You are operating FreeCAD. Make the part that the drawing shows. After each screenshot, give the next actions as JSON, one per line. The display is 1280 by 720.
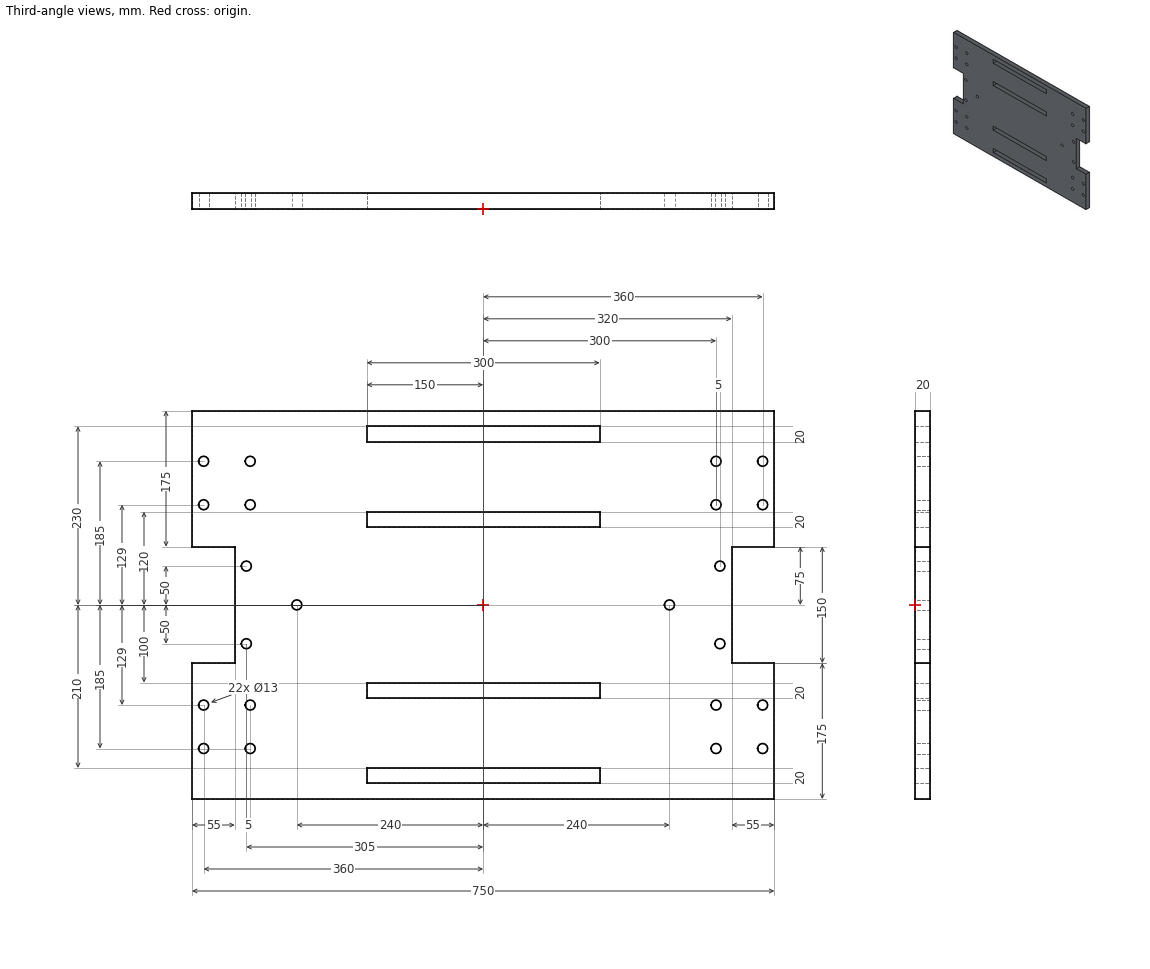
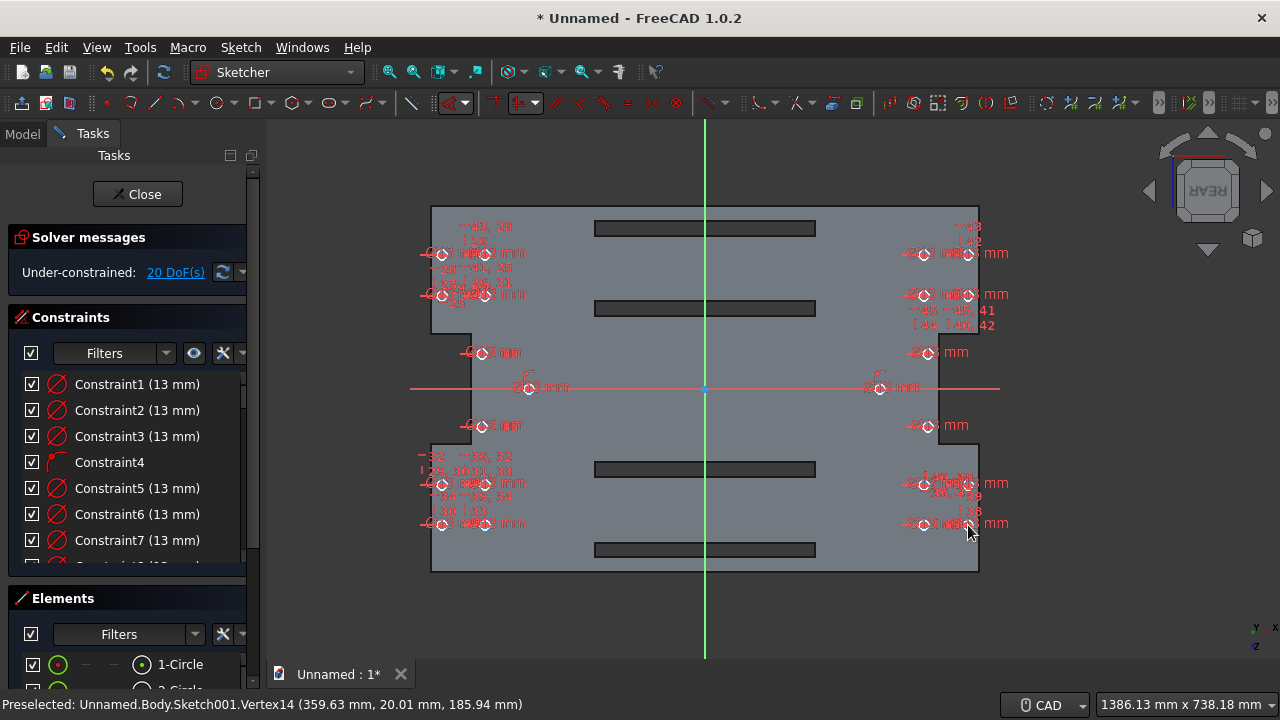
{"action": "left_click", "coordinate": [924, 525]}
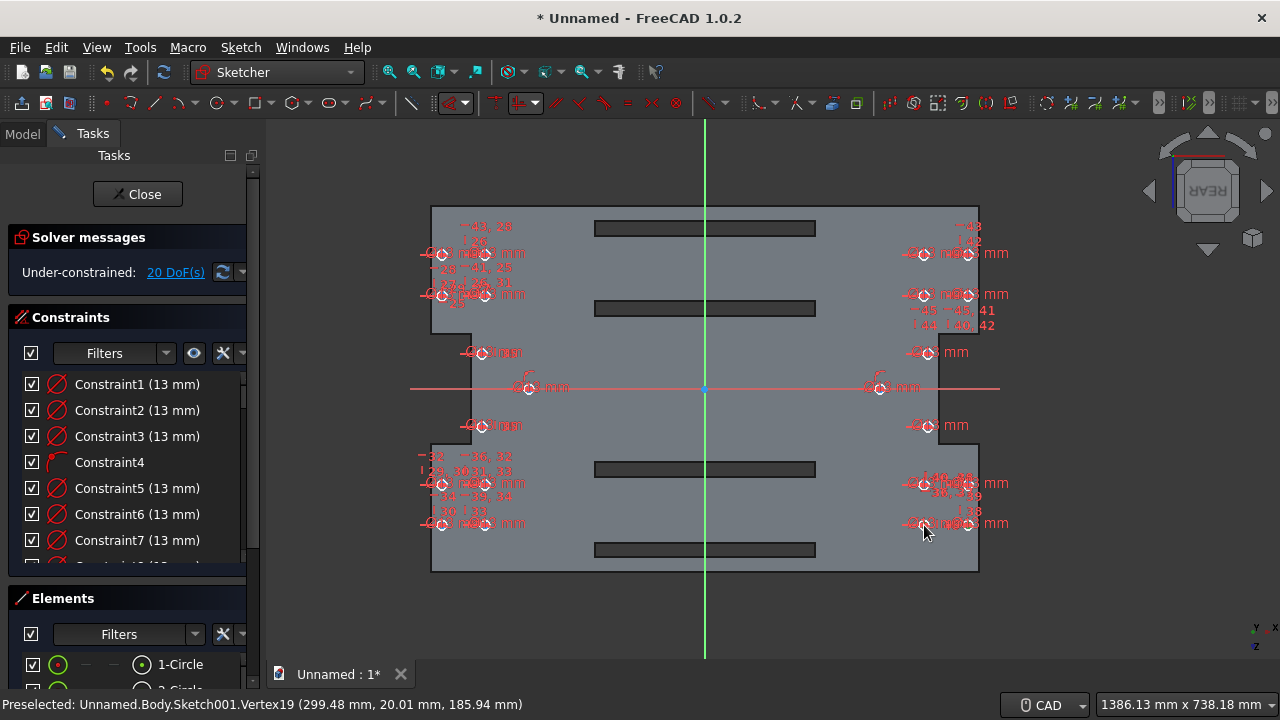
{"action": "left_click", "coordinate": [538, 104]}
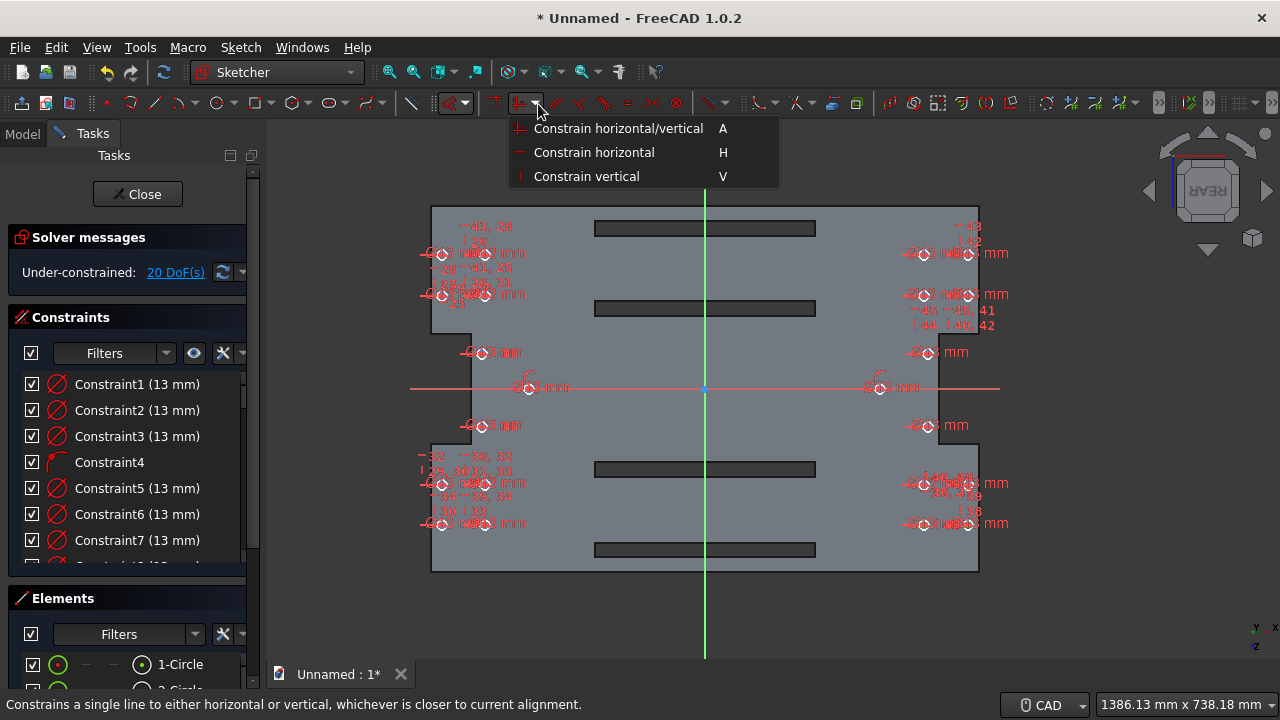
{"action": "left_click", "coordinate": [644, 152]}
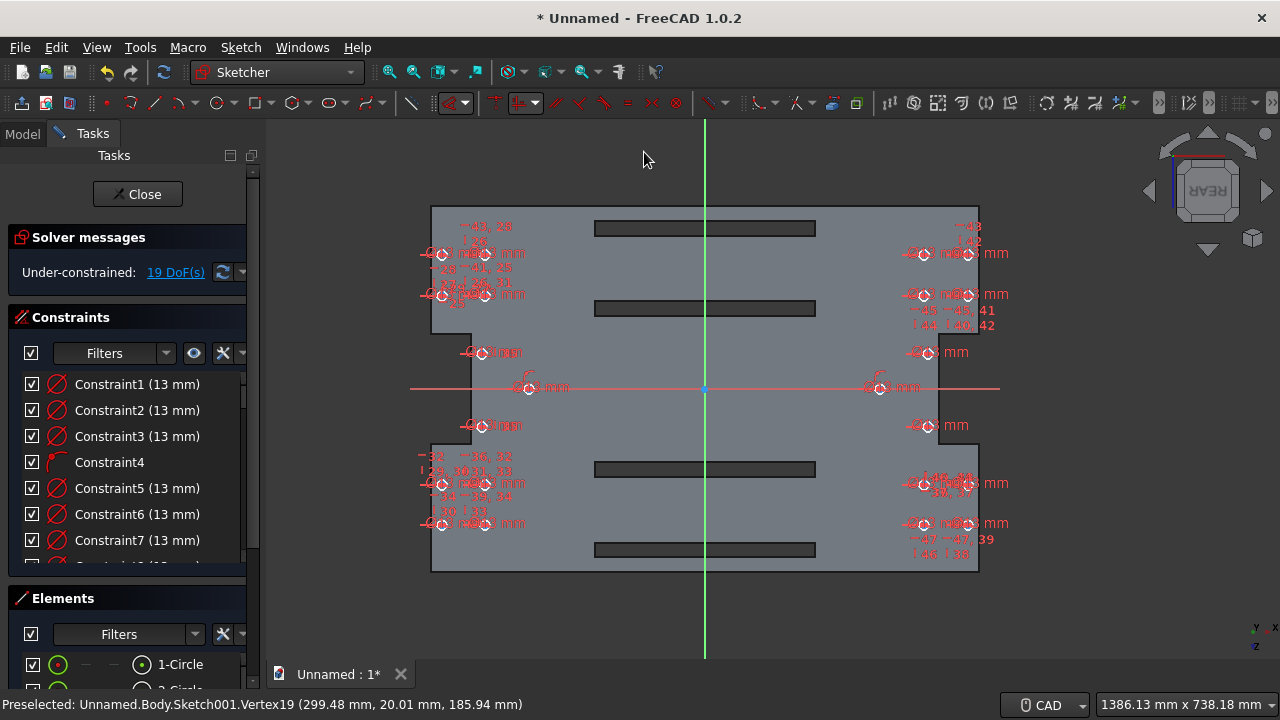
{"action": "left_click", "coordinate": [924, 296]}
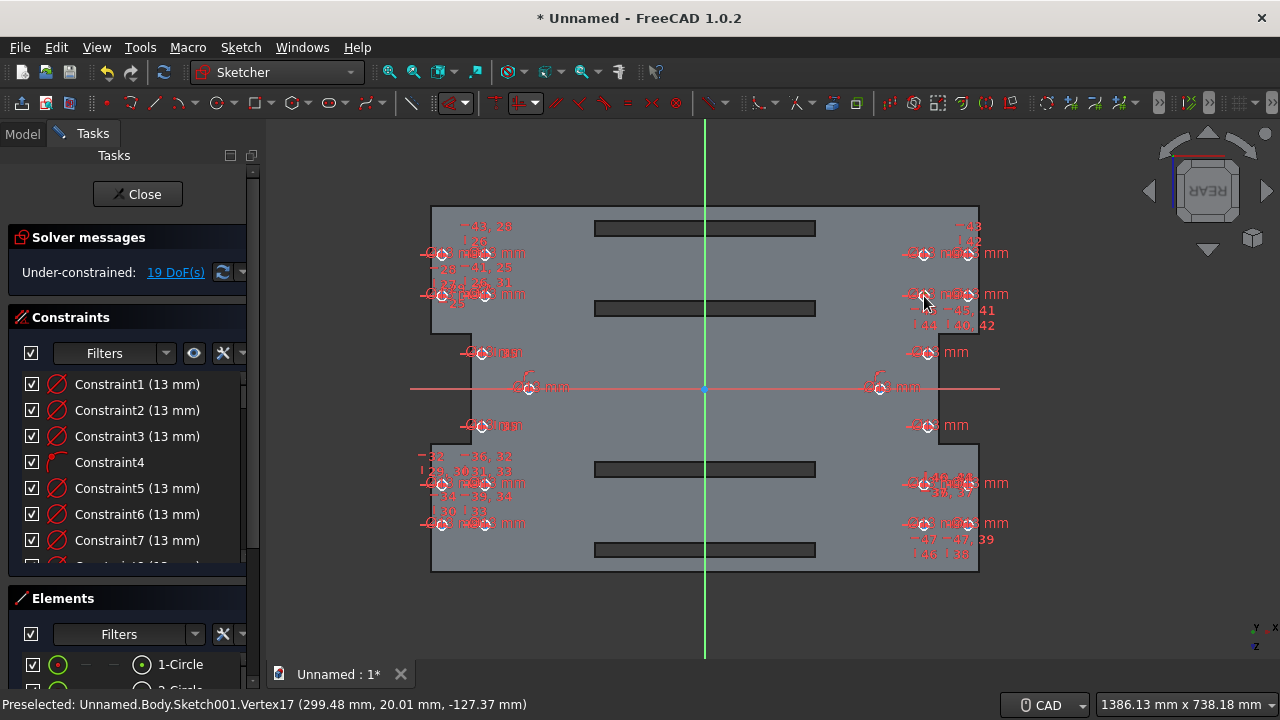
{"action": "left_click", "coordinate": [924, 255]}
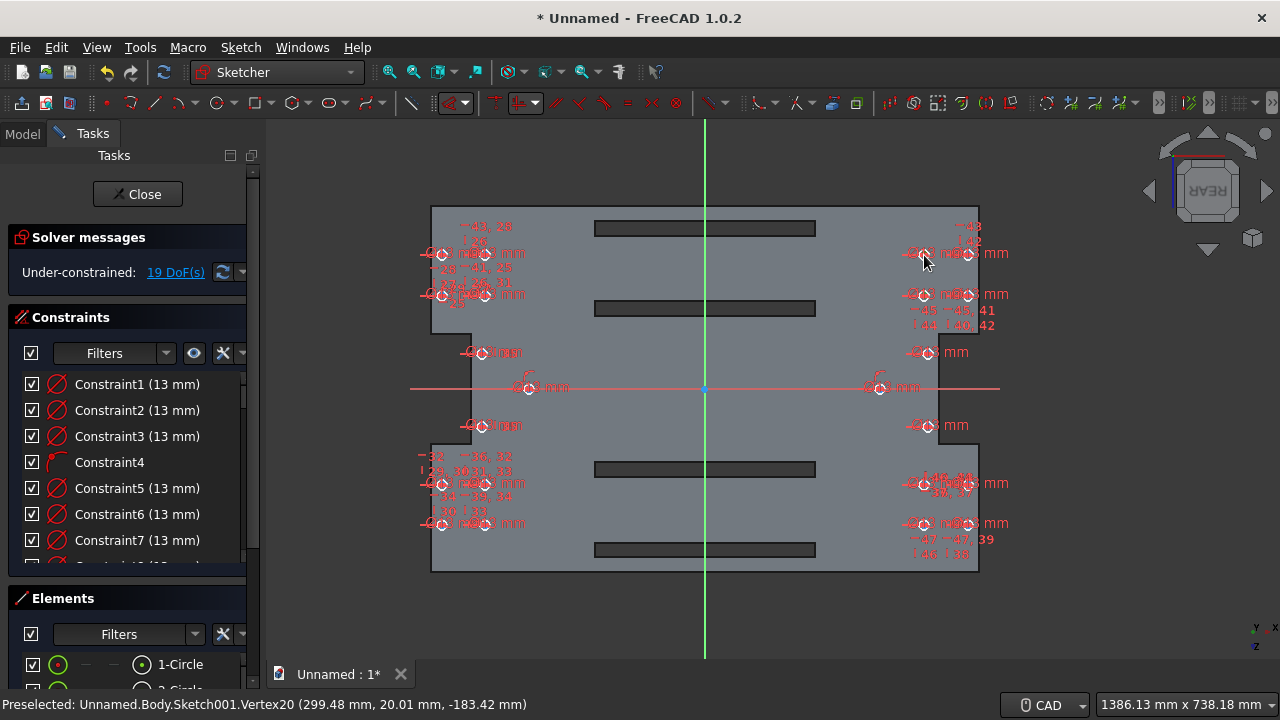
{"action": "left_click", "coordinate": [538, 104]}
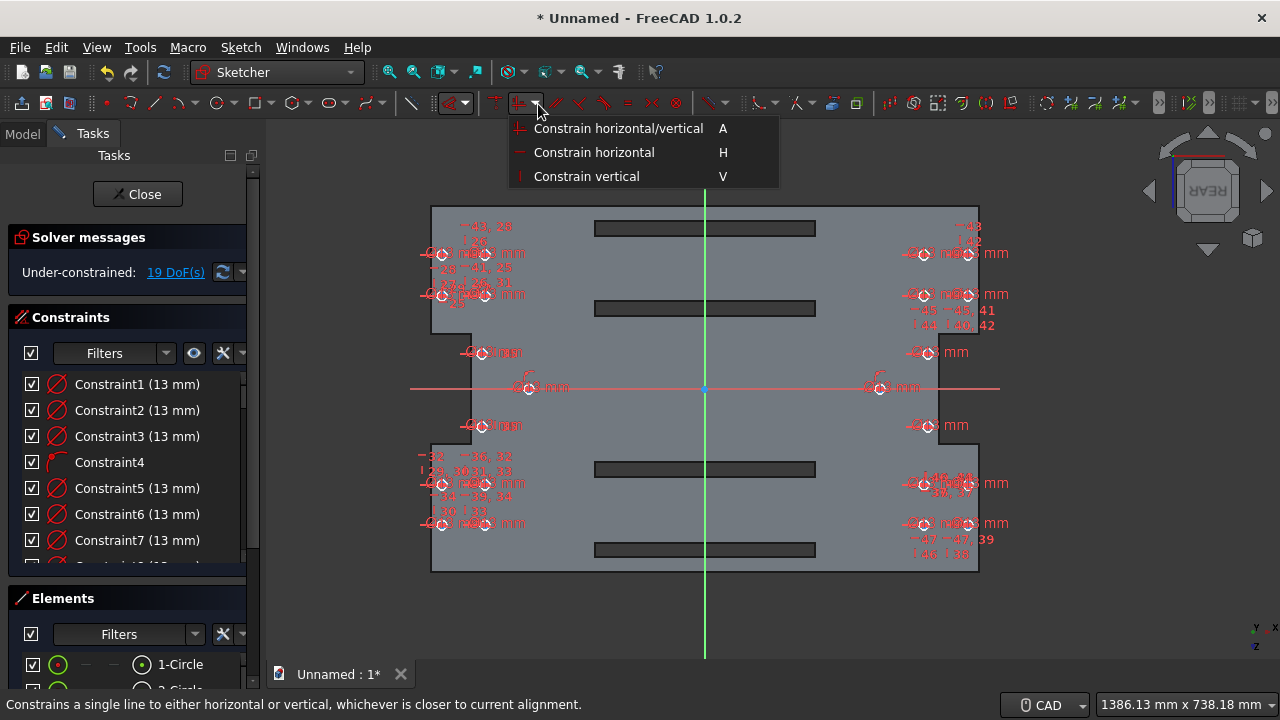
{"action": "left_click", "coordinate": [644, 176]}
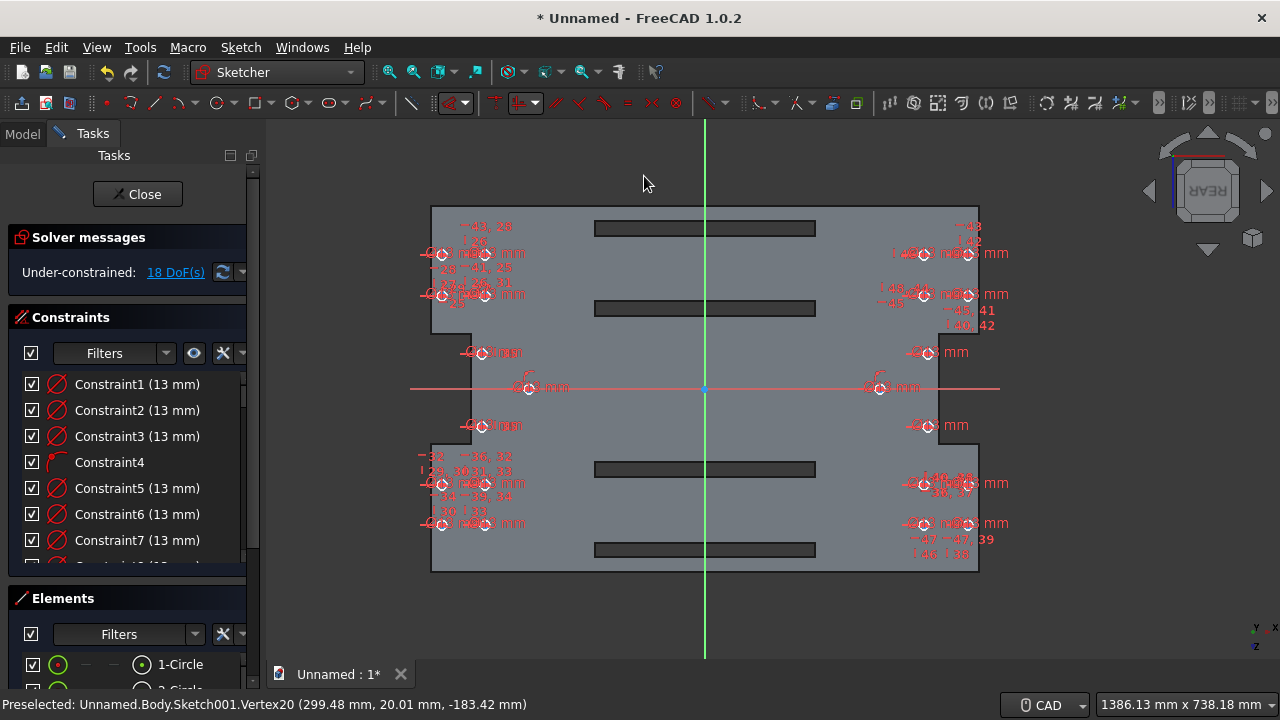
{"action": "left_click", "coordinate": [968, 255]}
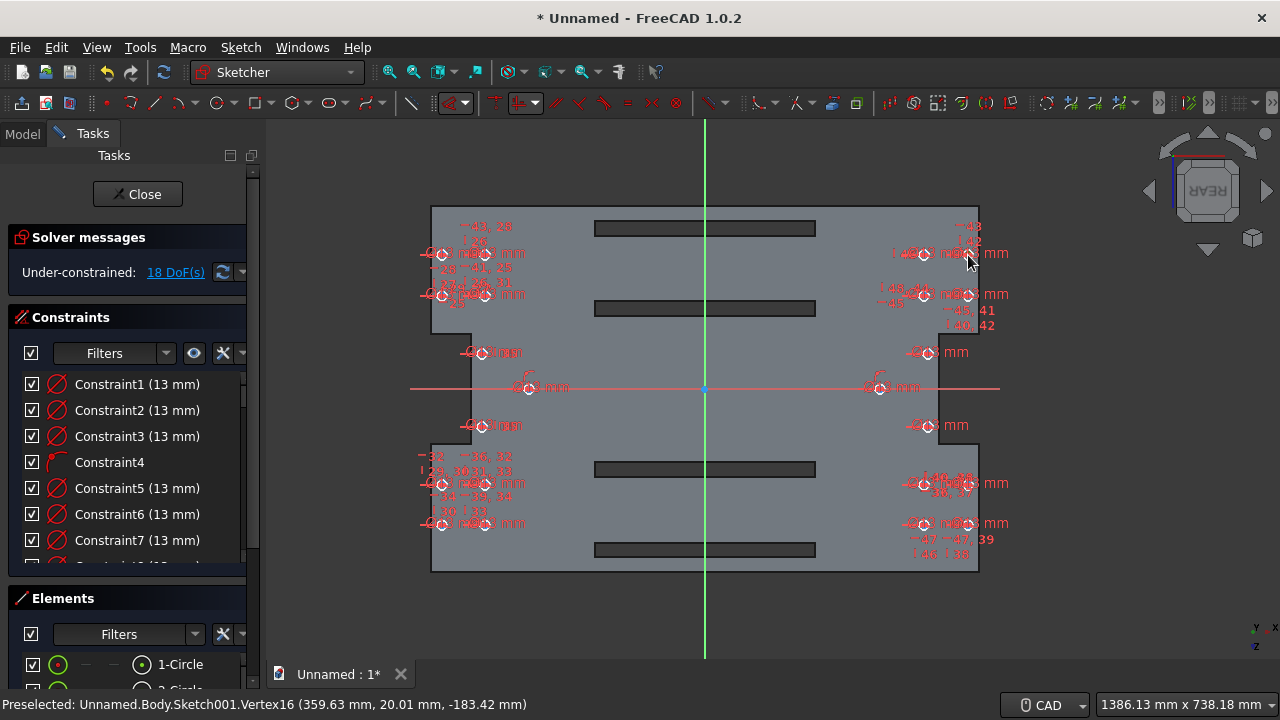
{"action": "left_click", "coordinate": [924, 255]}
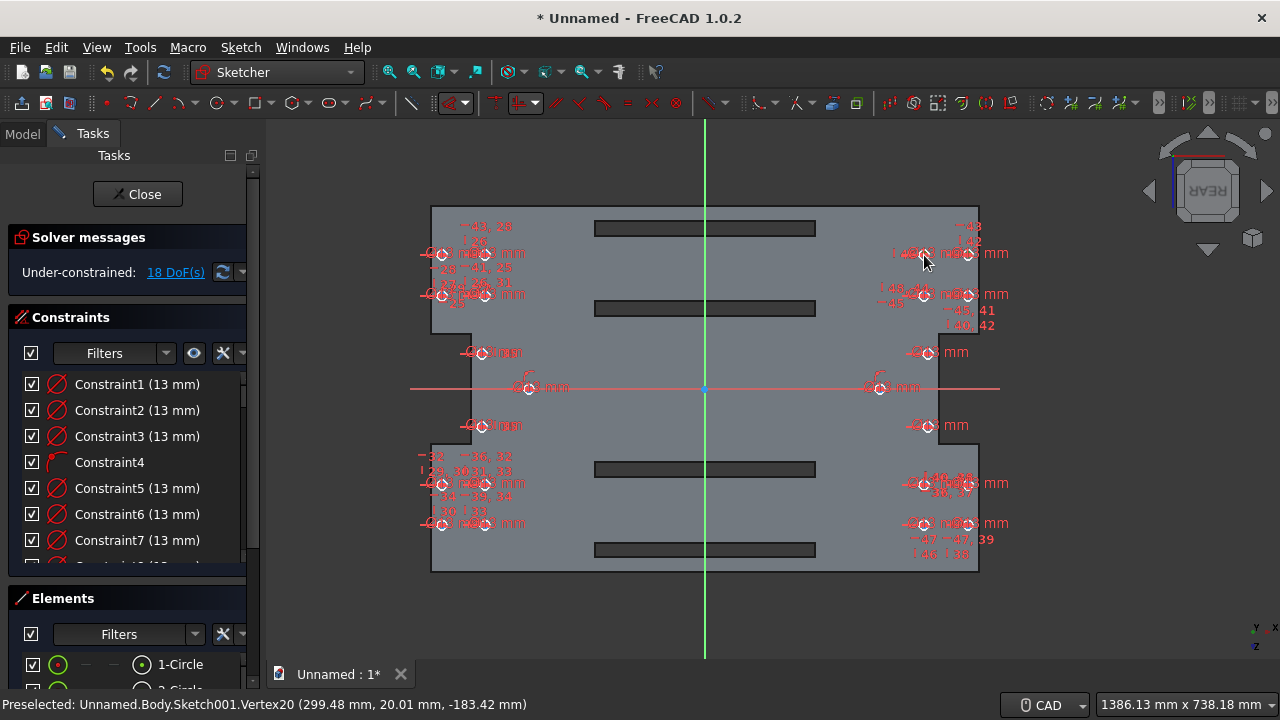
{"action": "left_click", "coordinate": [538, 104]}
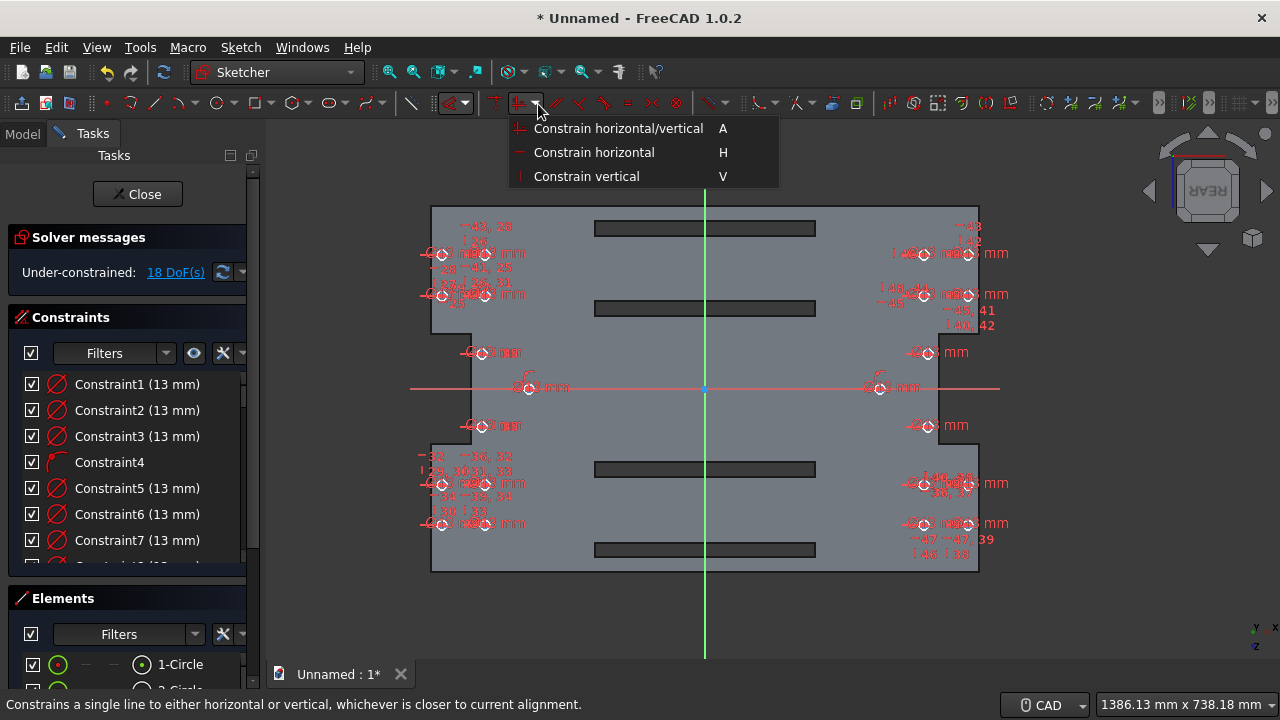
{"action": "left_click", "coordinate": [644, 152]}